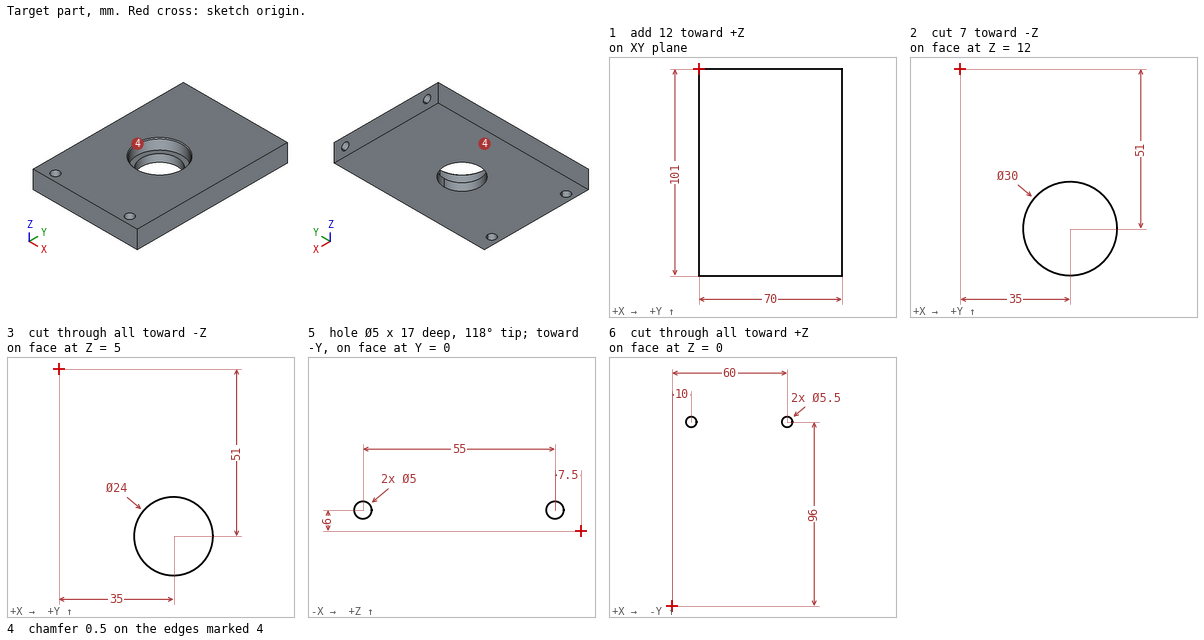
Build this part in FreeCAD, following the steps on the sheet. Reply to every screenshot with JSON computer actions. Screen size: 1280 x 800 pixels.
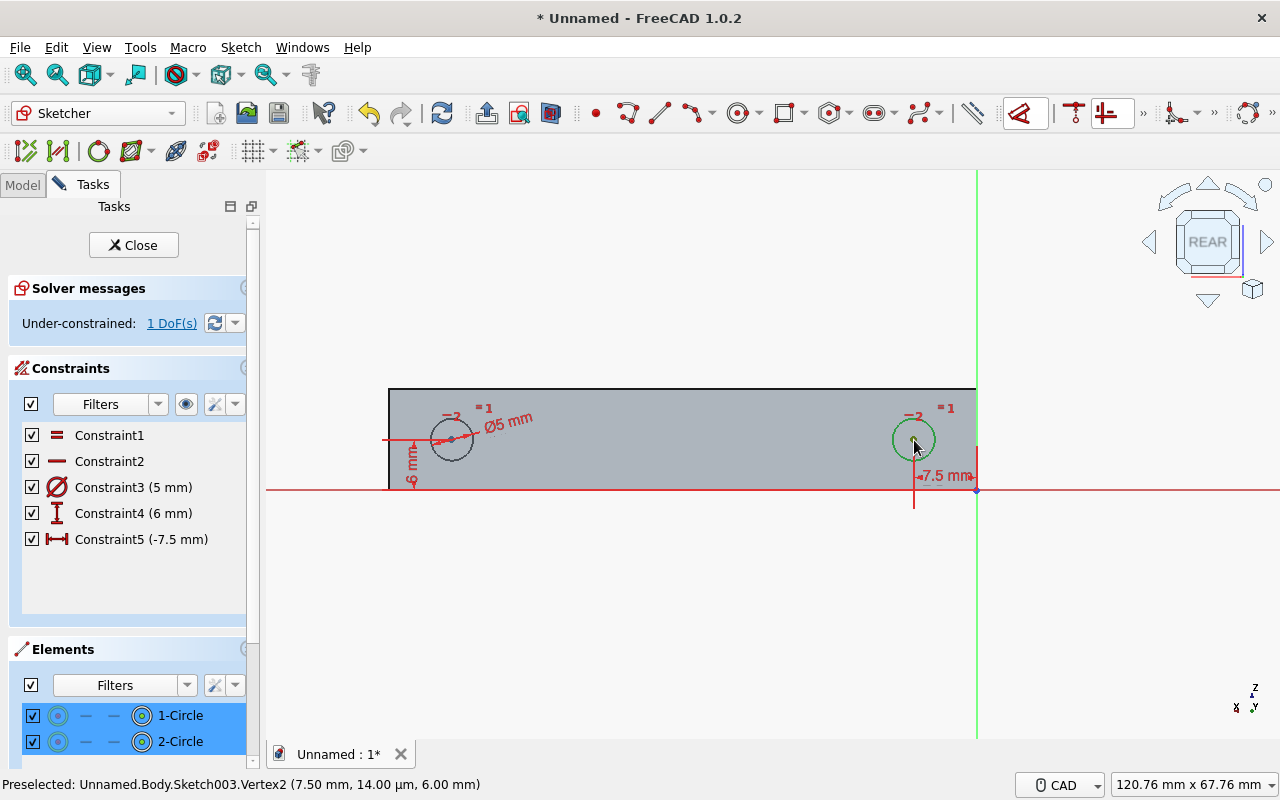
{"action": "left_click", "coordinate": [1042, 114]}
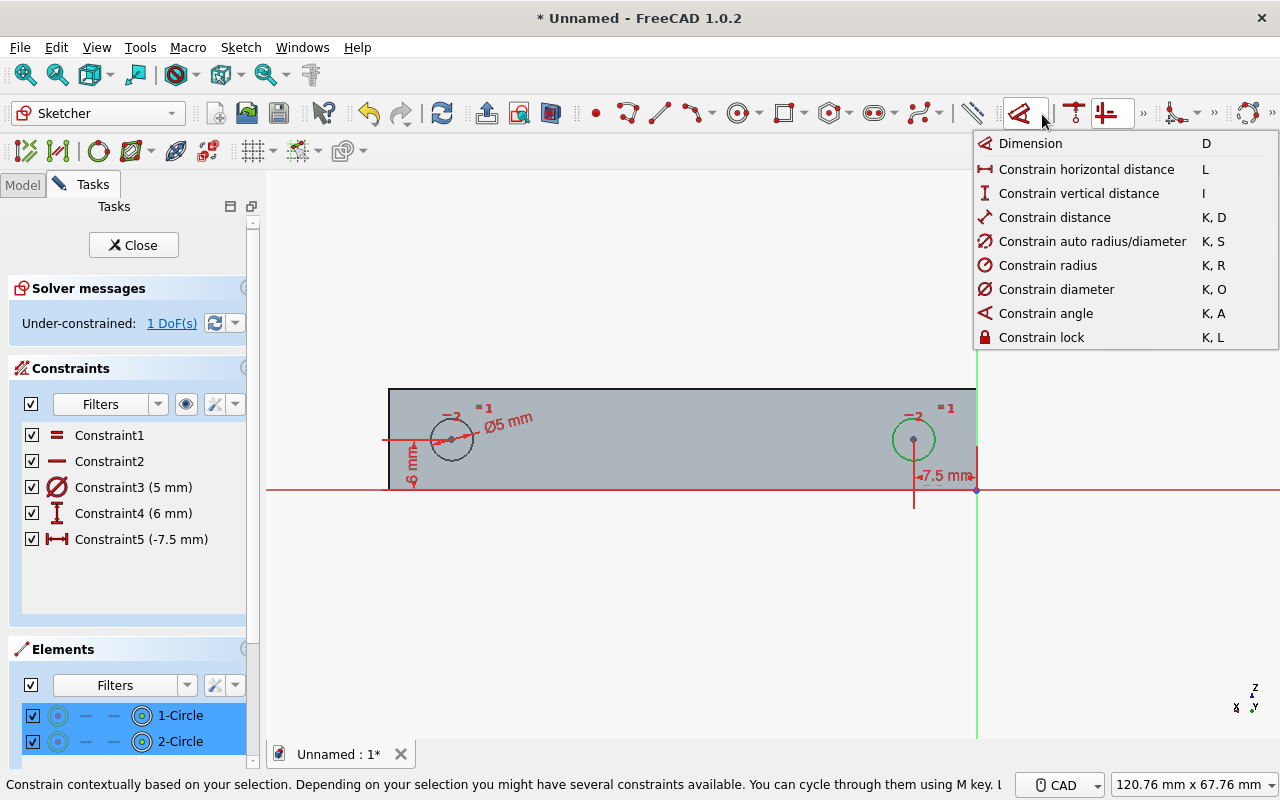
{"action": "left_click", "coordinate": [1126, 169]}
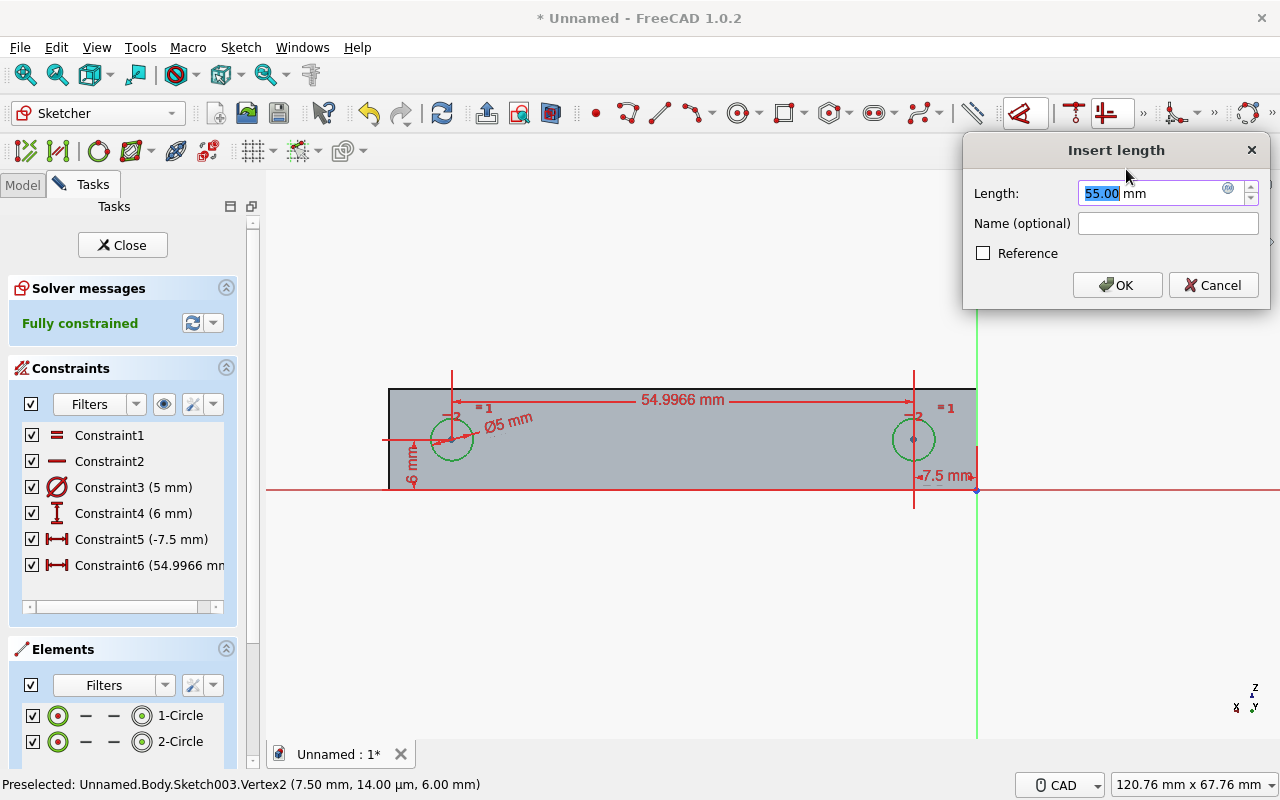
{"action": "type", "text": "55"}
{"action": "key", "text": "Return"}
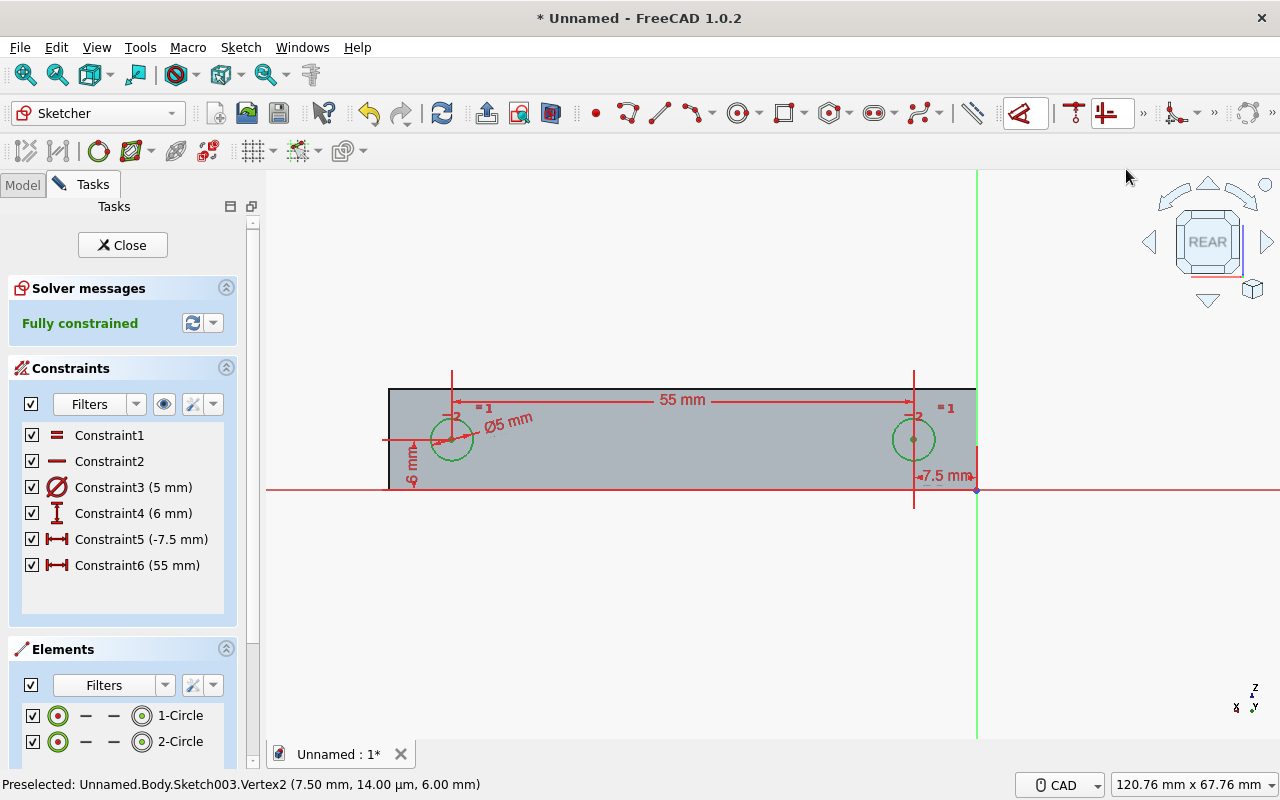
{"action": "left_click", "coordinate": [123, 245]}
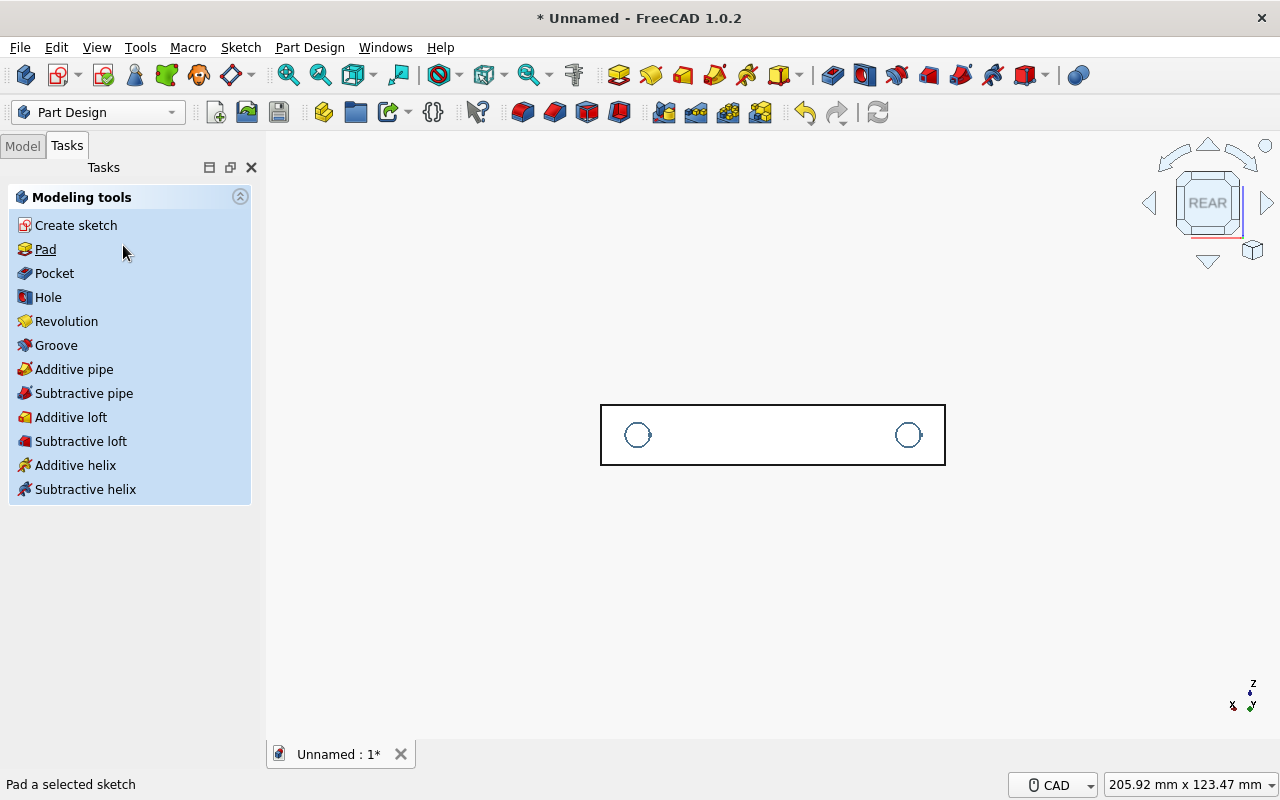
{"action": "left_click", "coordinate": [866, 76]}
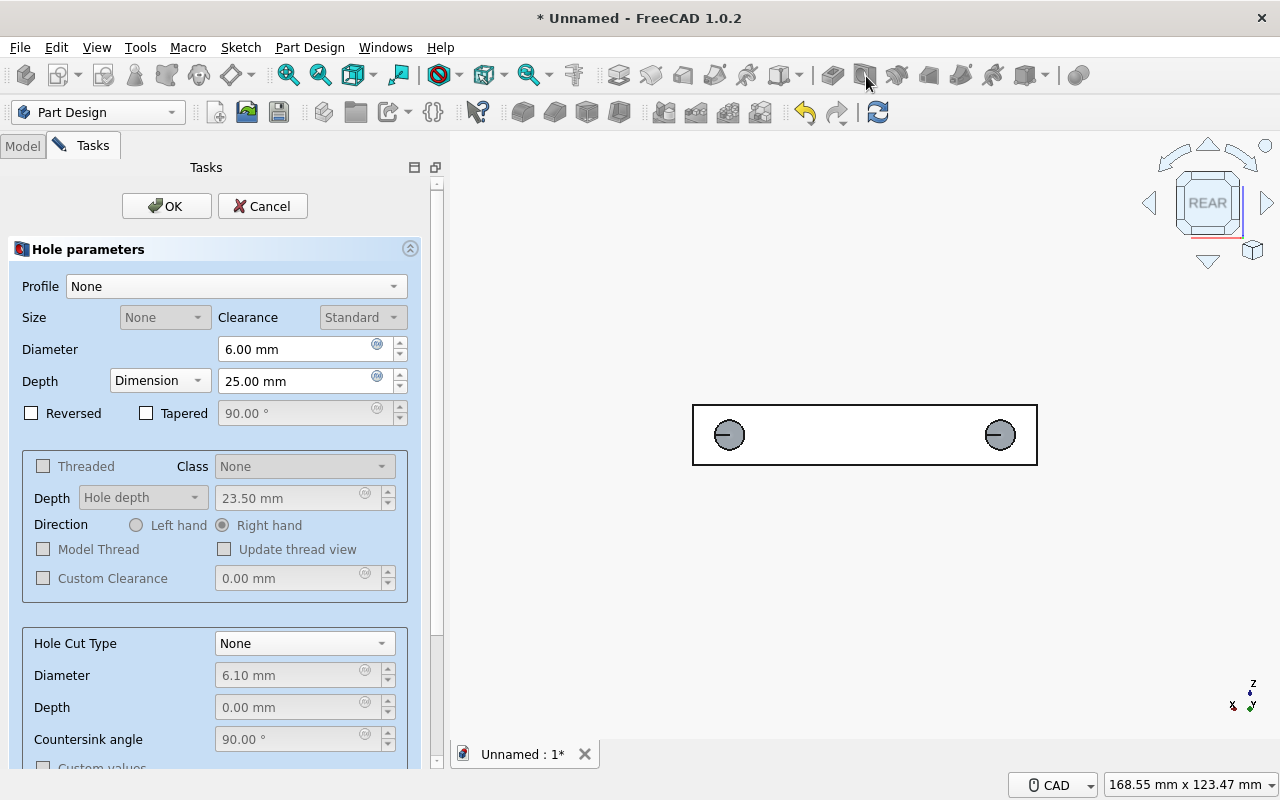
{"action": "triple_click", "coordinate": [305, 349]}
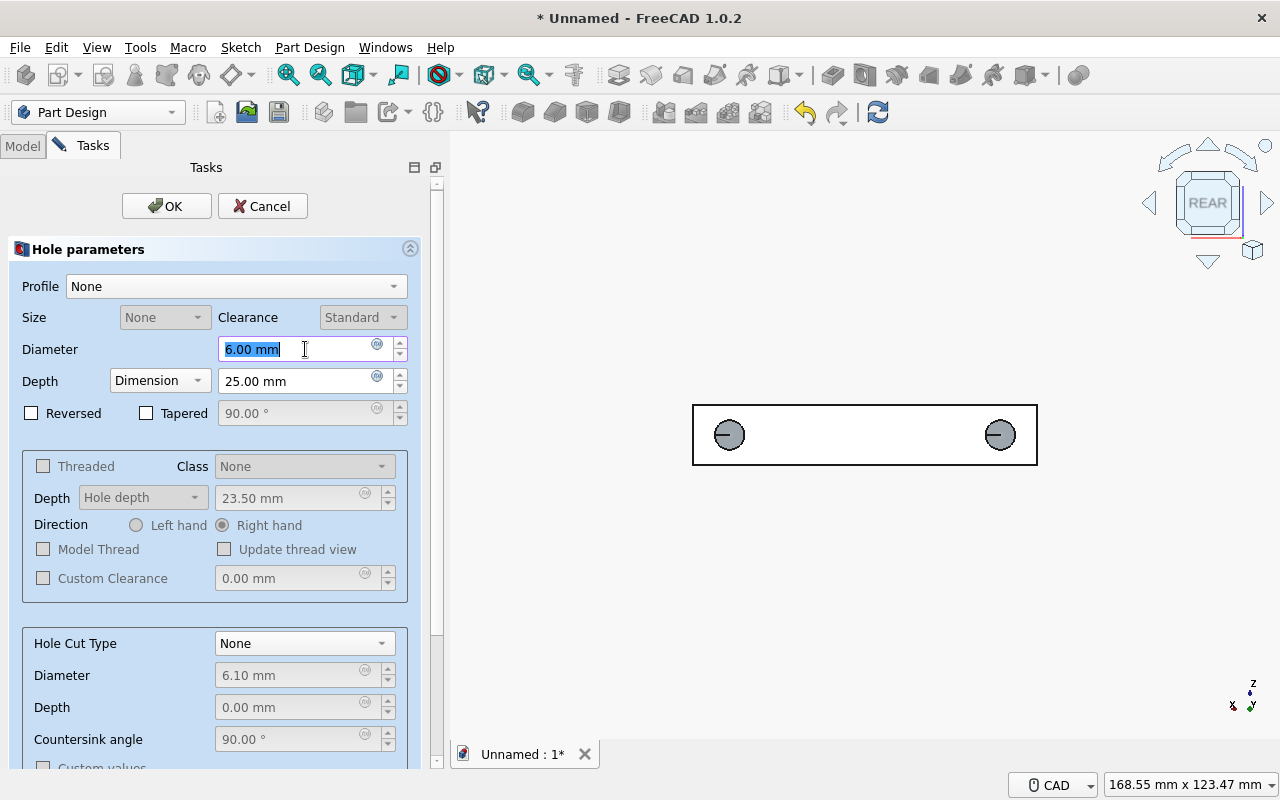
{"action": "type", "text": "5"}
{"action": "key", "text": "Tab"}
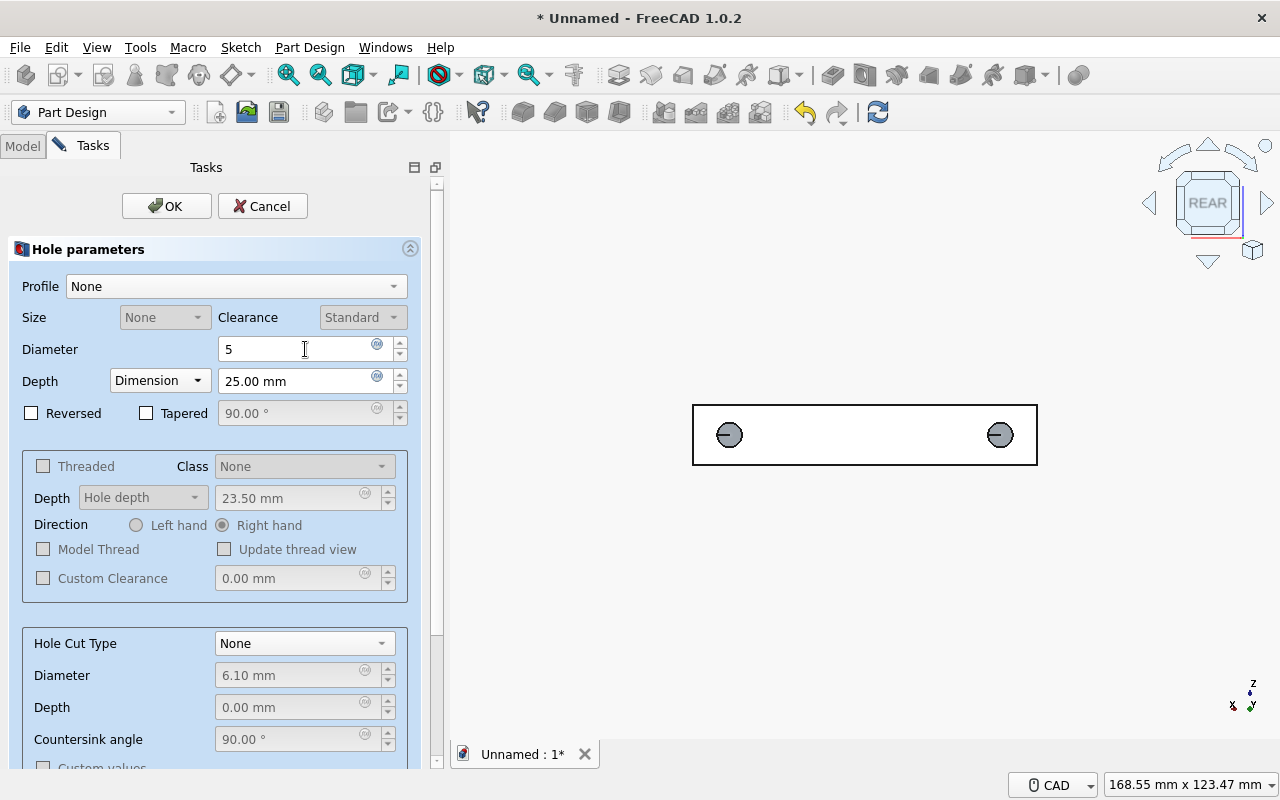
{"action": "triple_click", "coordinate": [305, 381]}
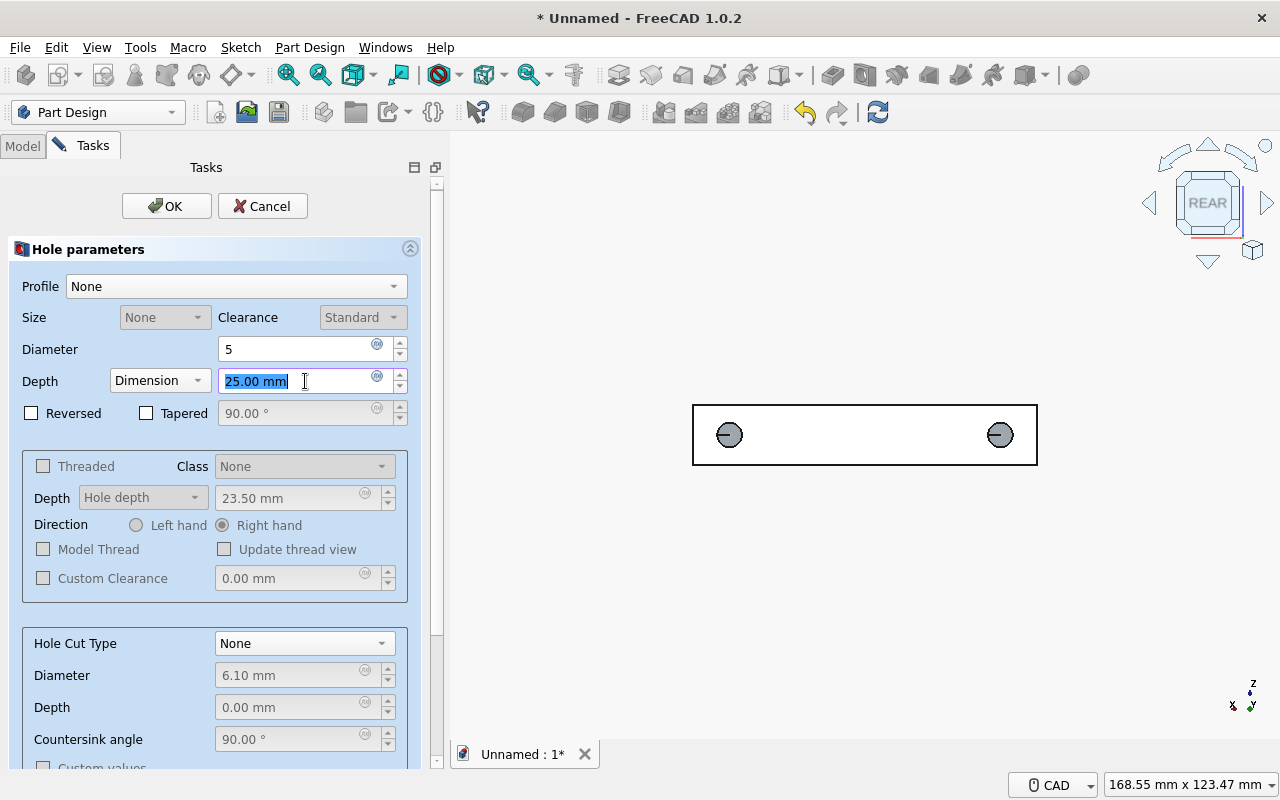
{"action": "type", "text": "17"}
{"action": "key", "text": "Tab"}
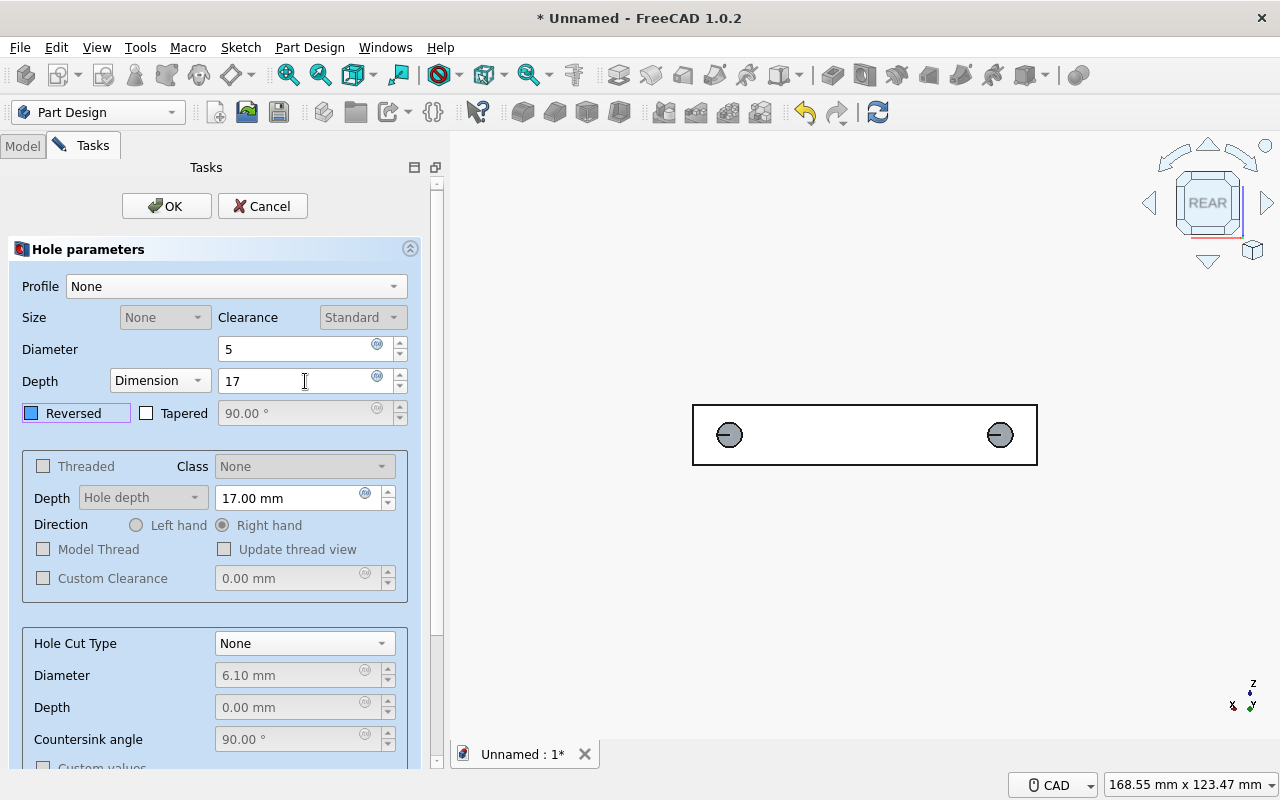
{"action": "left_click", "coordinate": [167, 206]}